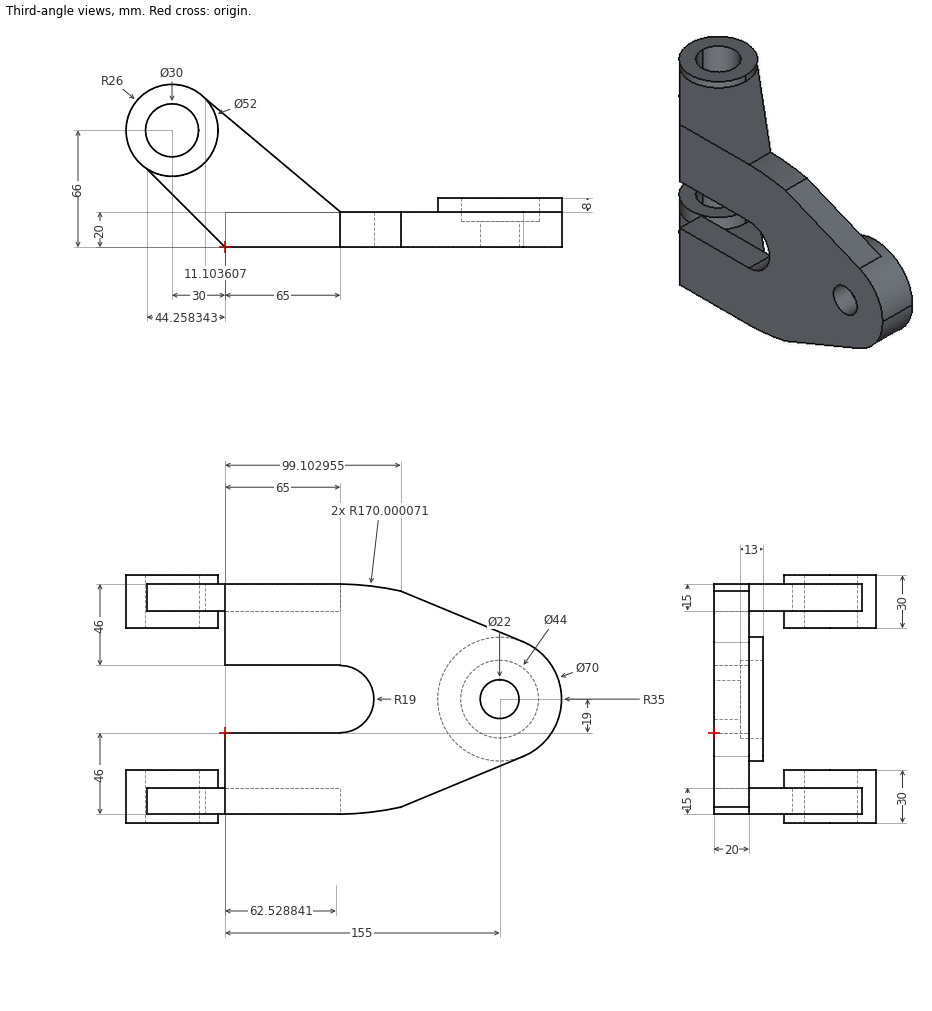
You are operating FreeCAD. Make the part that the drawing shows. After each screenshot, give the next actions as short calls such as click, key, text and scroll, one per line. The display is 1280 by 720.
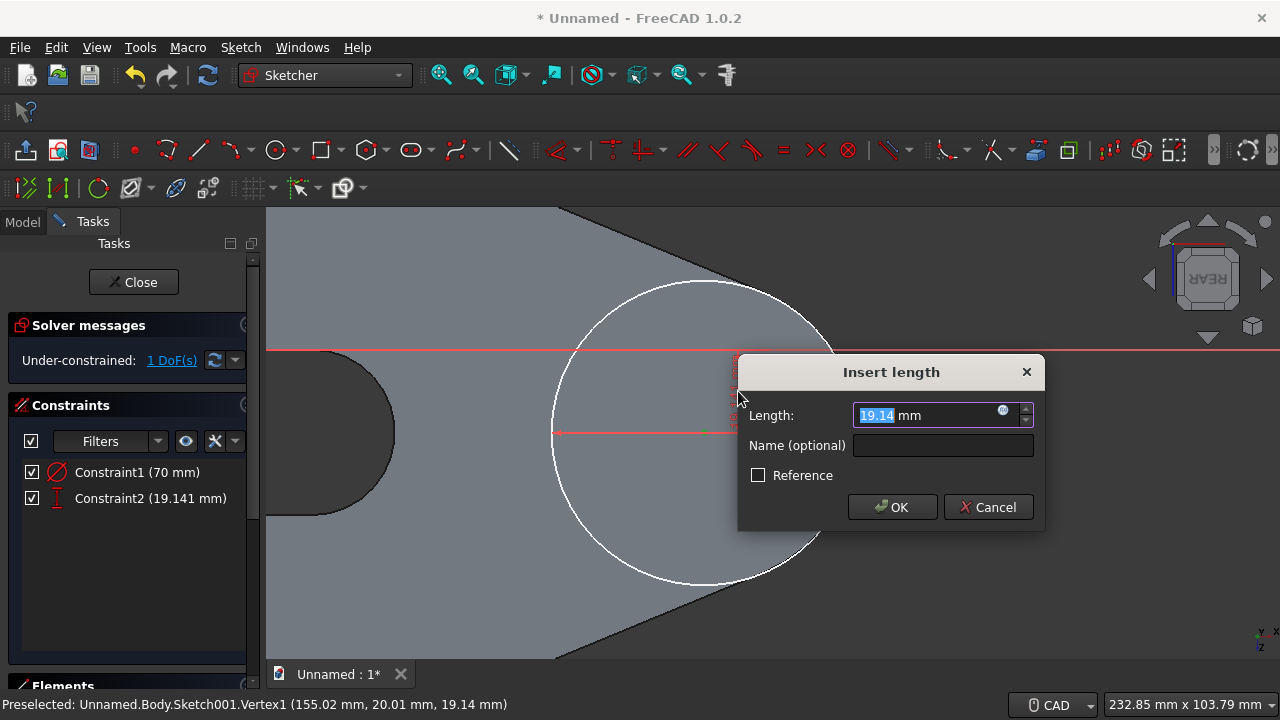
text(19)
key(Return)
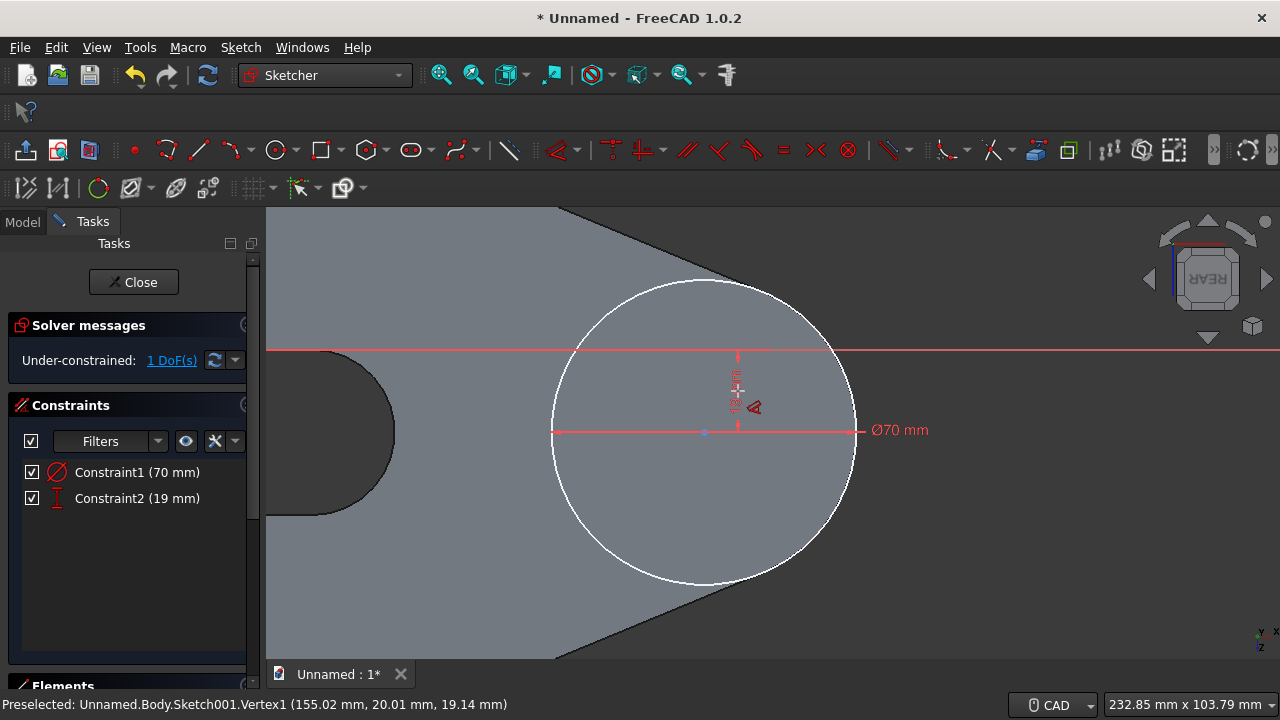
click(704, 432)
click(499, 316)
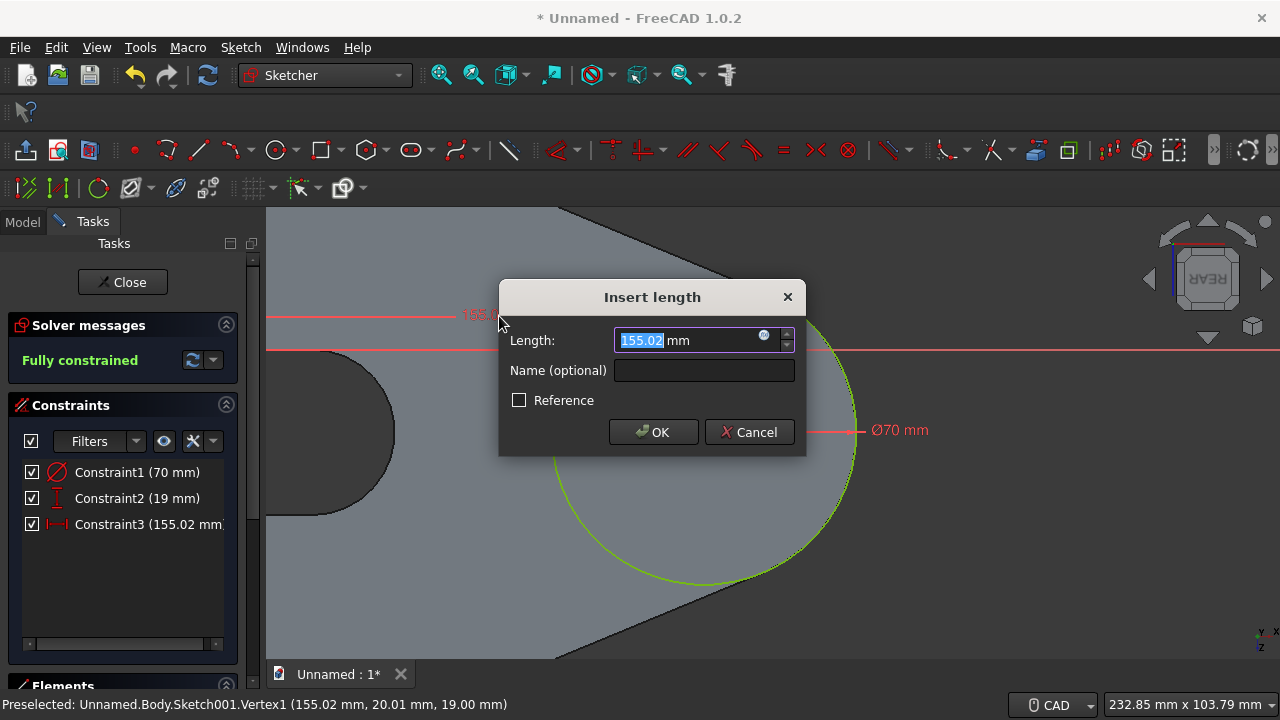
text(155)
key(Return)
key(Escape)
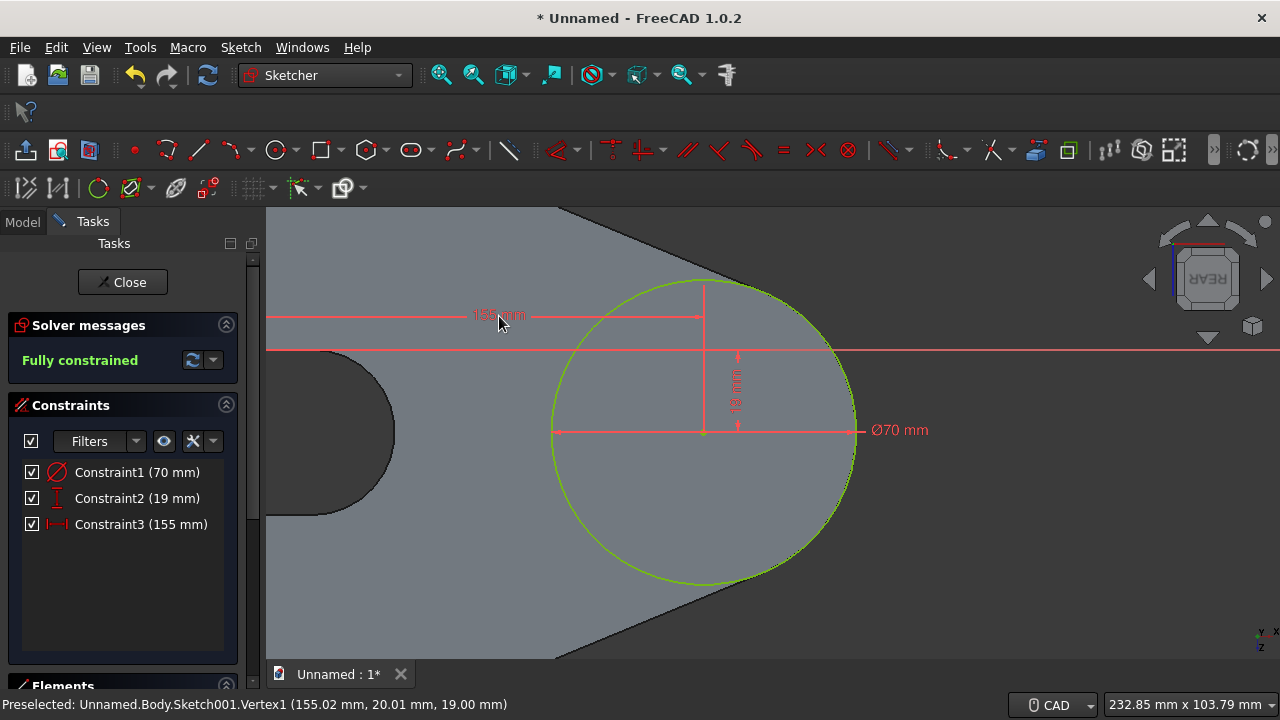
click(123, 282)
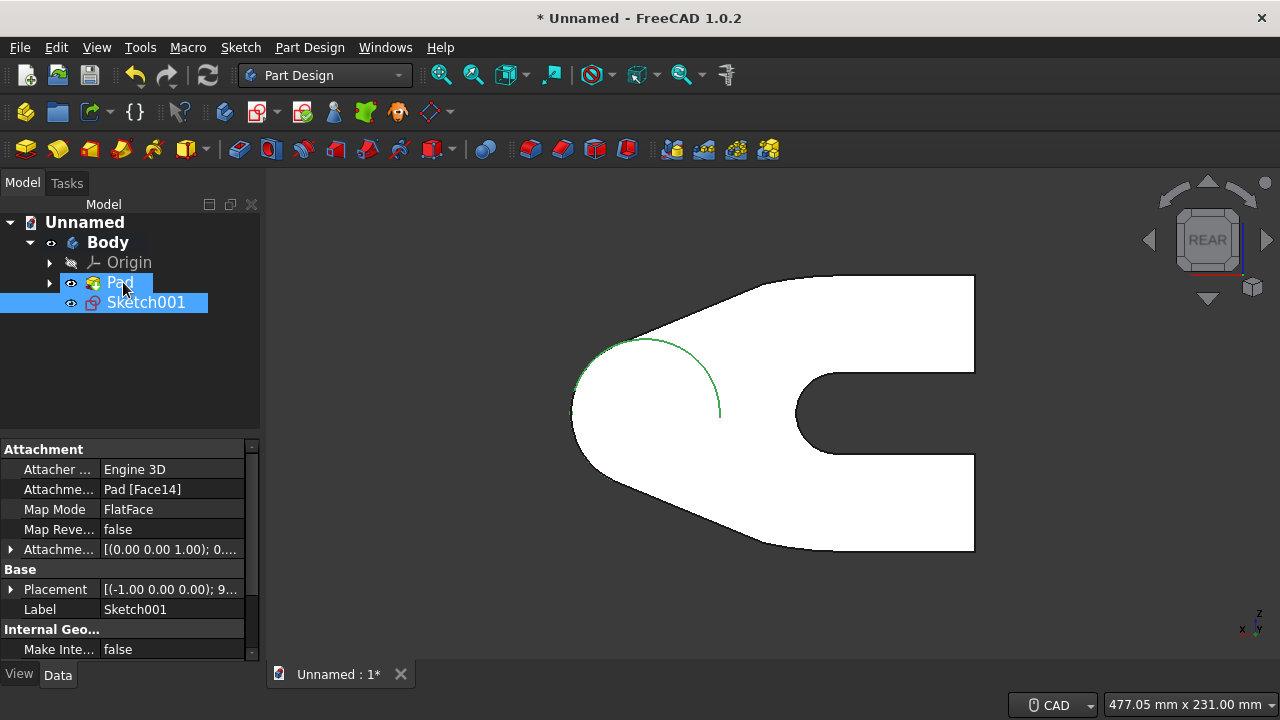
click(26, 150)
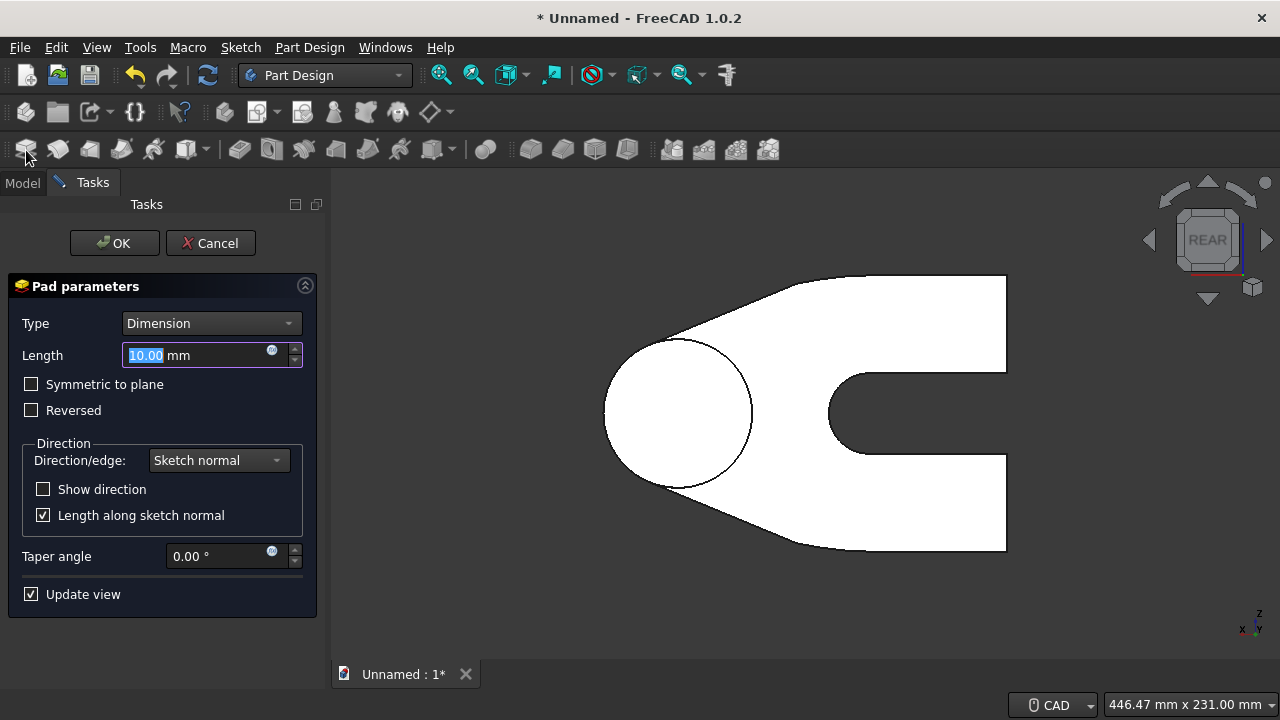
text(8)
key(Tab)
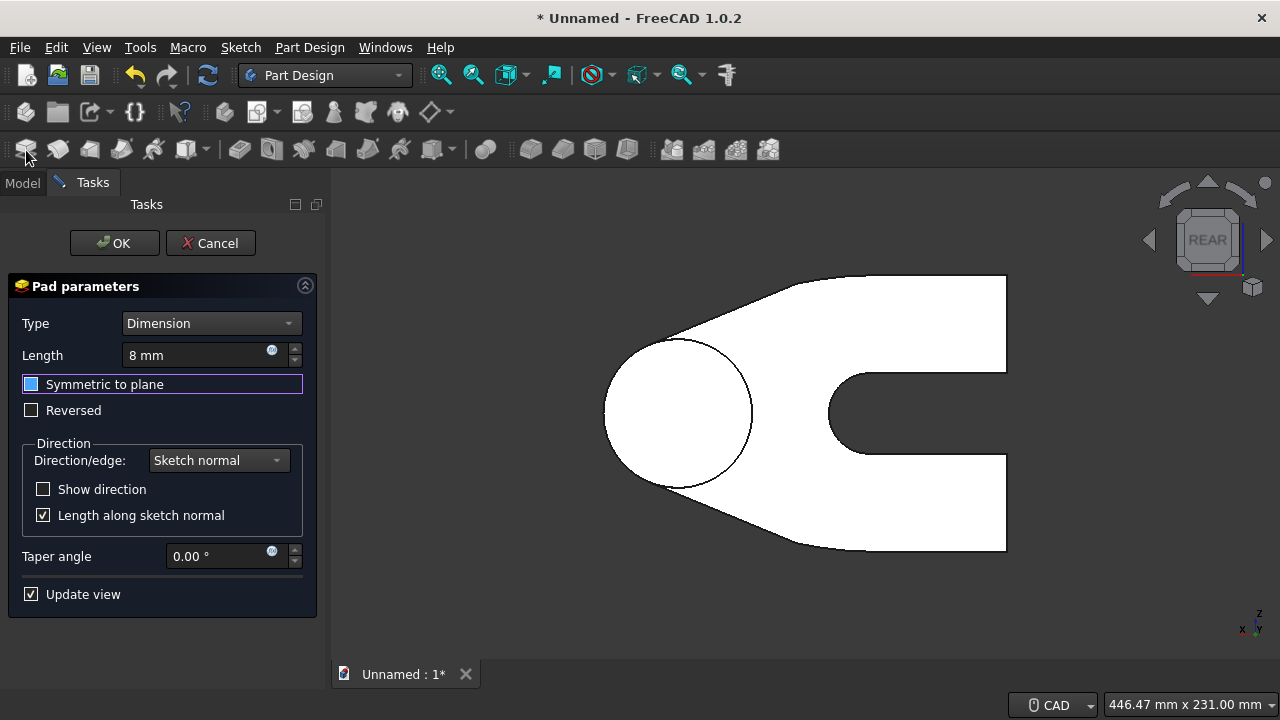
click(115, 243)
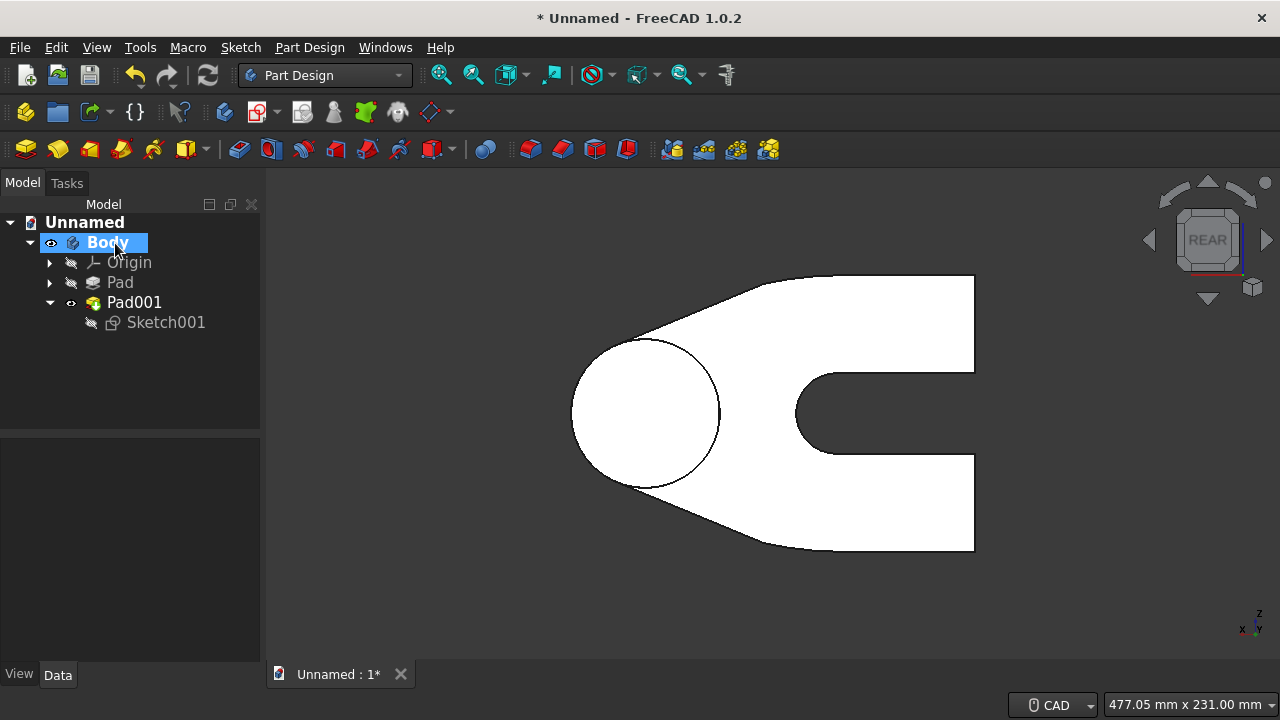
key(0)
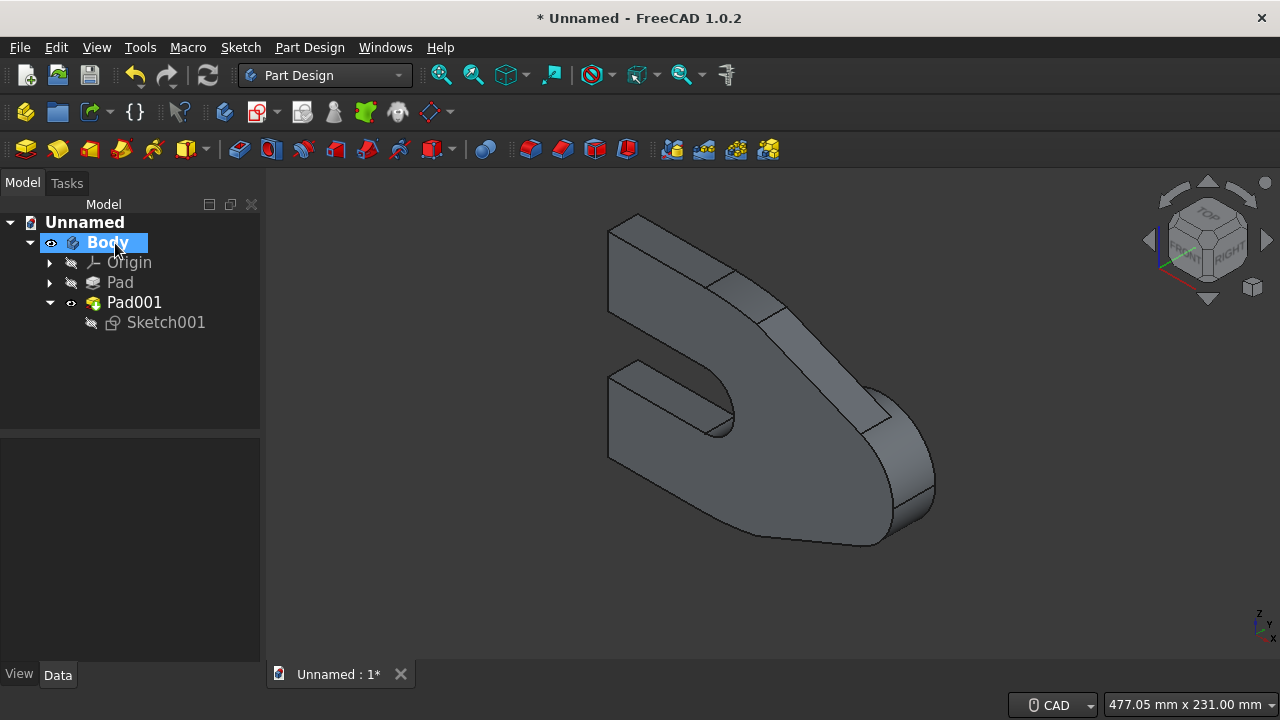
click(700, 266)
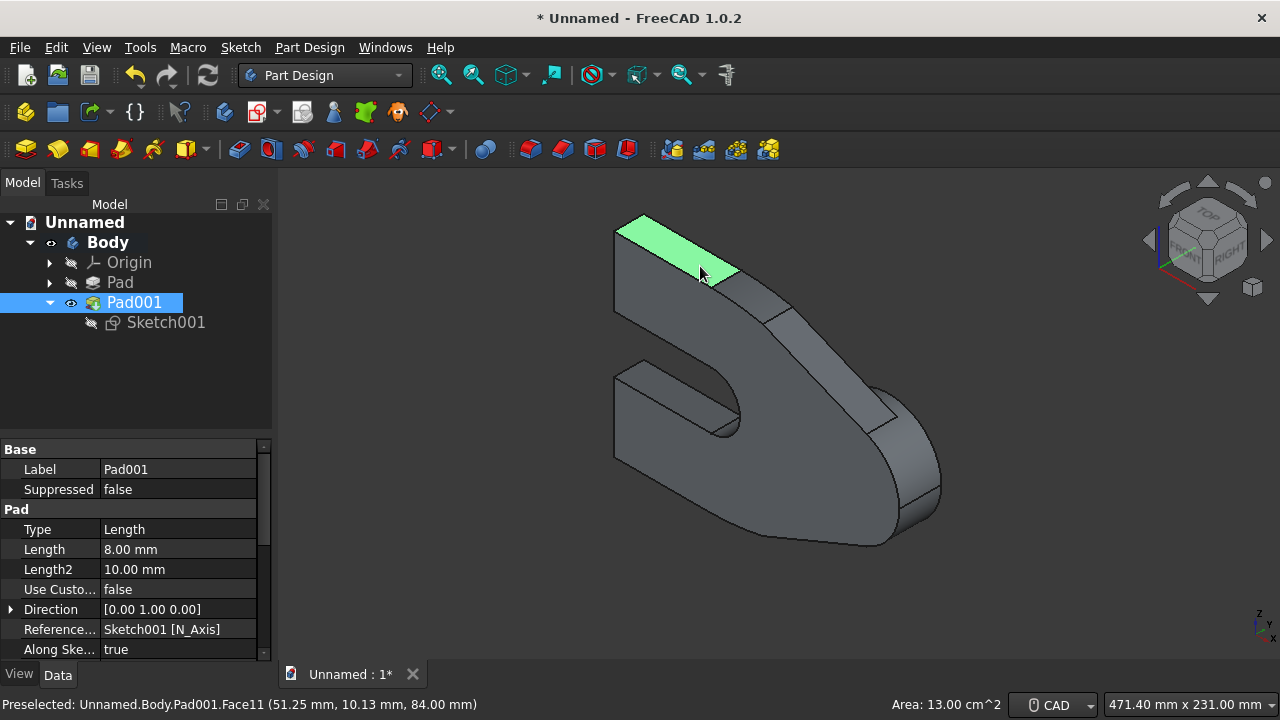
click(258, 112)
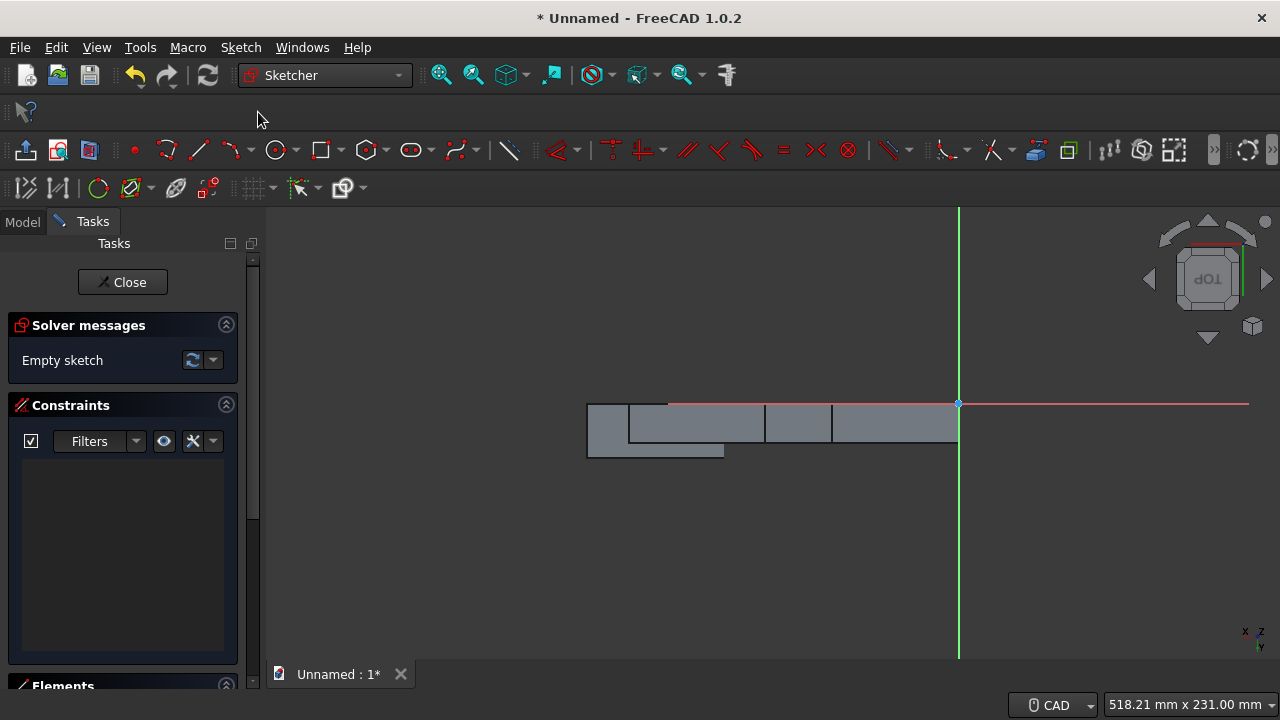
scroll(1115, 550, up, 3)